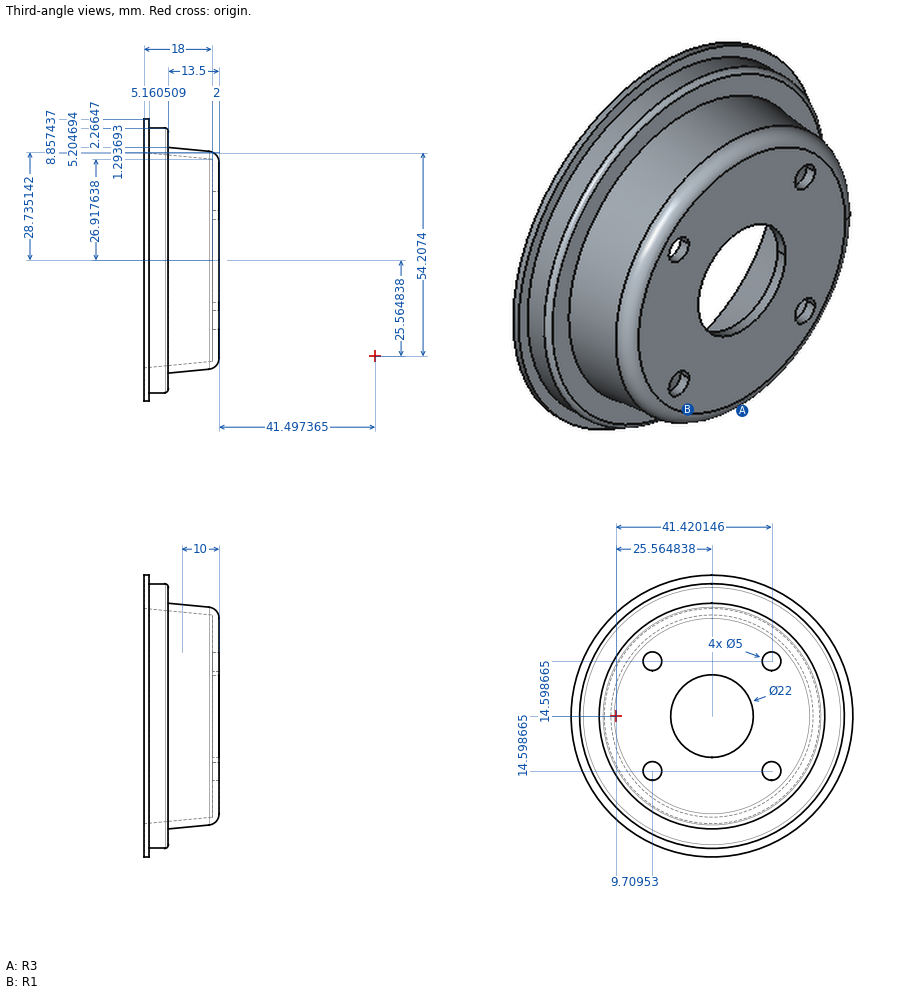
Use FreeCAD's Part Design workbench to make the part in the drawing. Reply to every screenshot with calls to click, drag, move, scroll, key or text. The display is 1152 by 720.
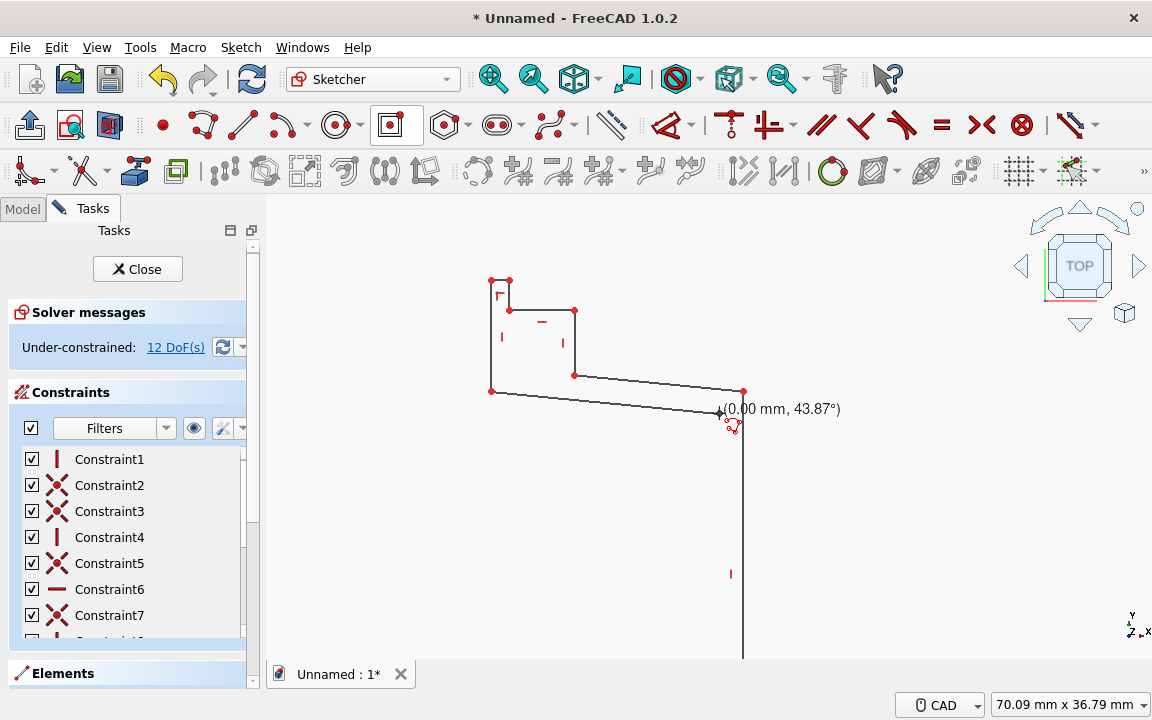
scroll(501, 280, down, 5)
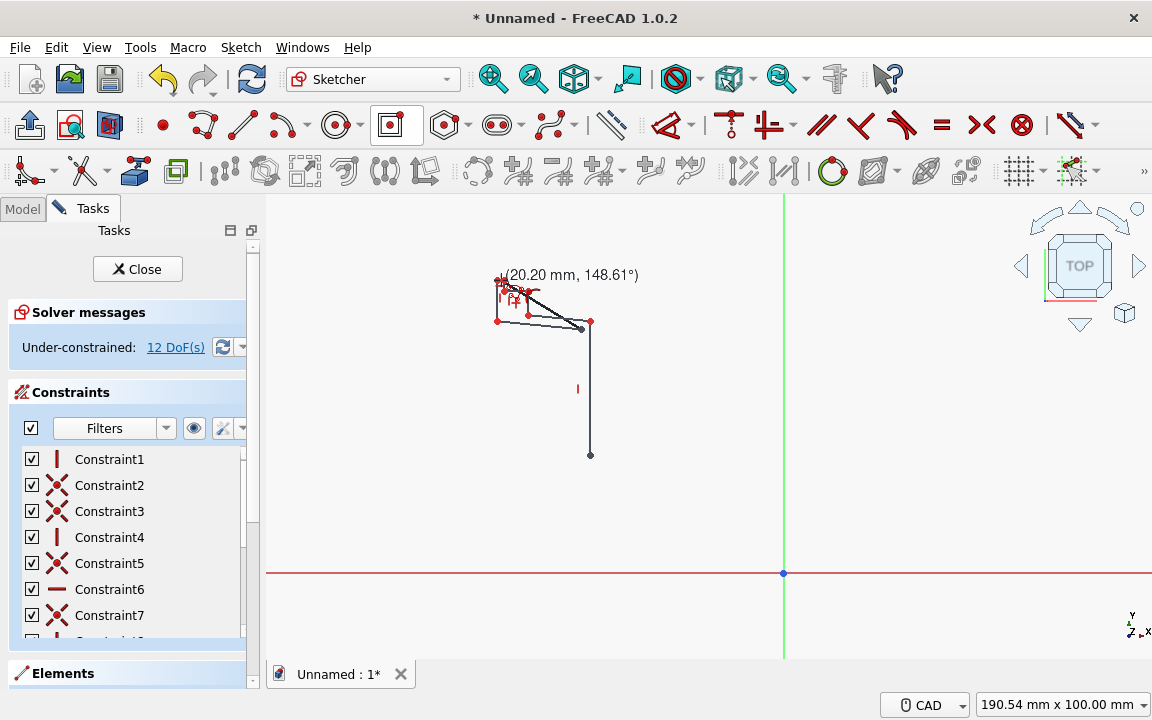
scroll(581, 454, up, 3)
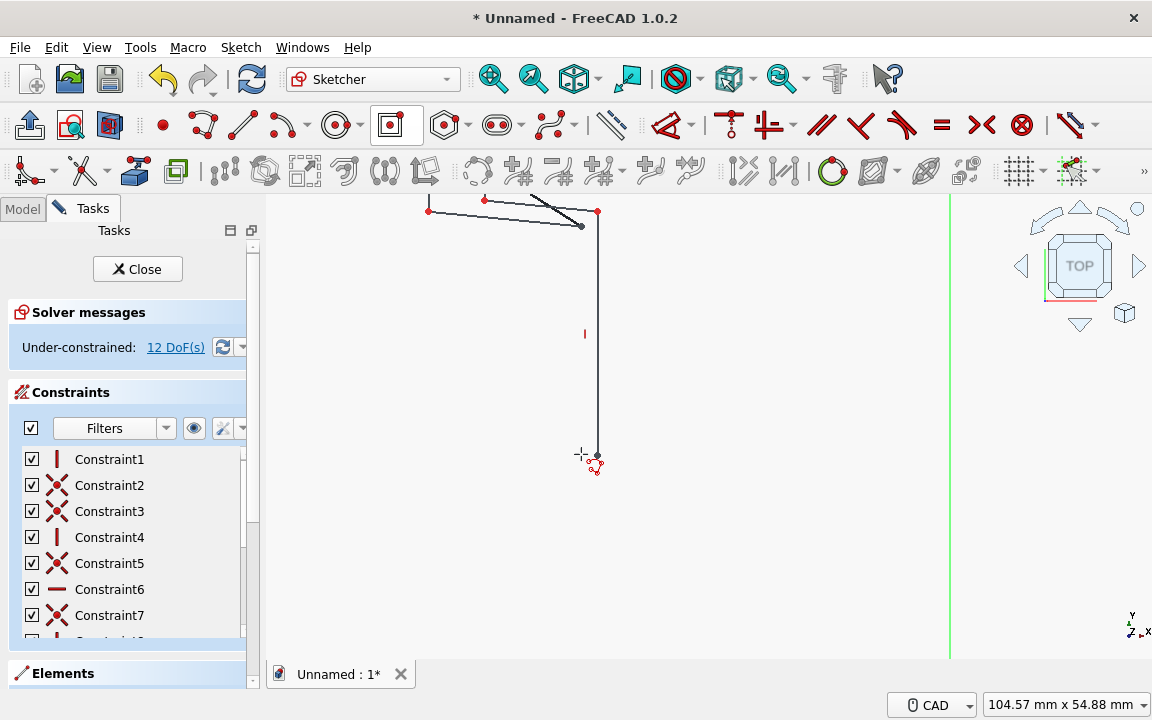
click(581, 454)
click(598, 456)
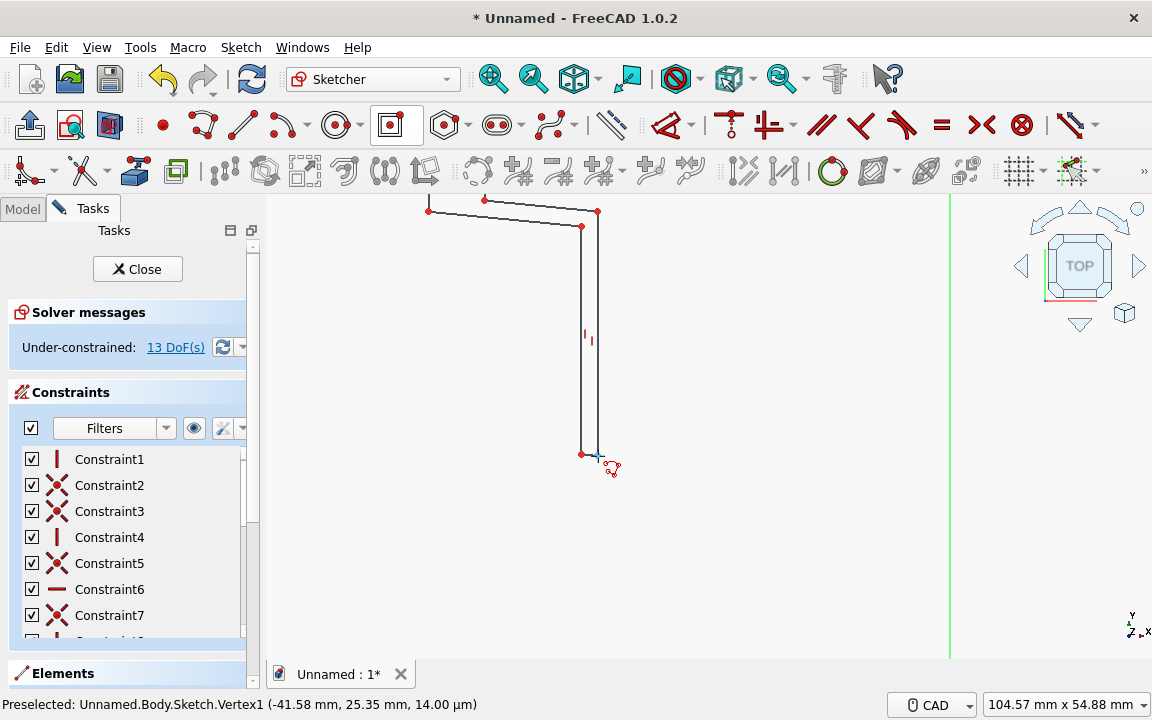
click(244, 126)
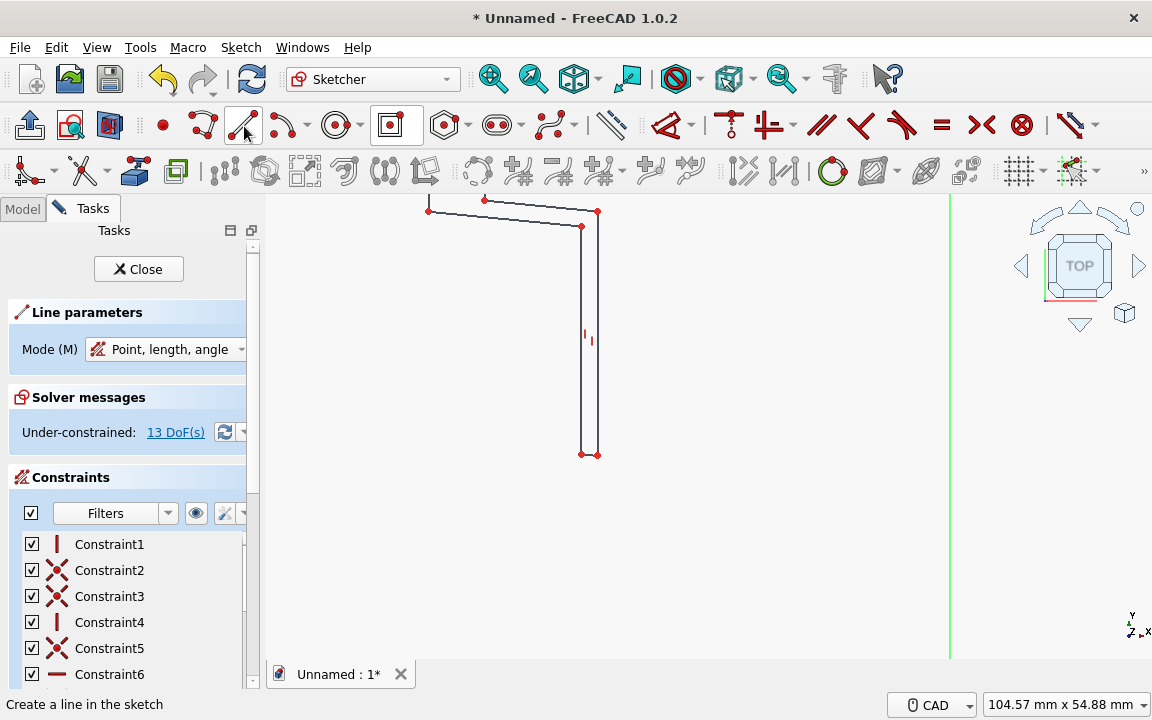
click(615, 454)
click(666, 454)
key(Escape)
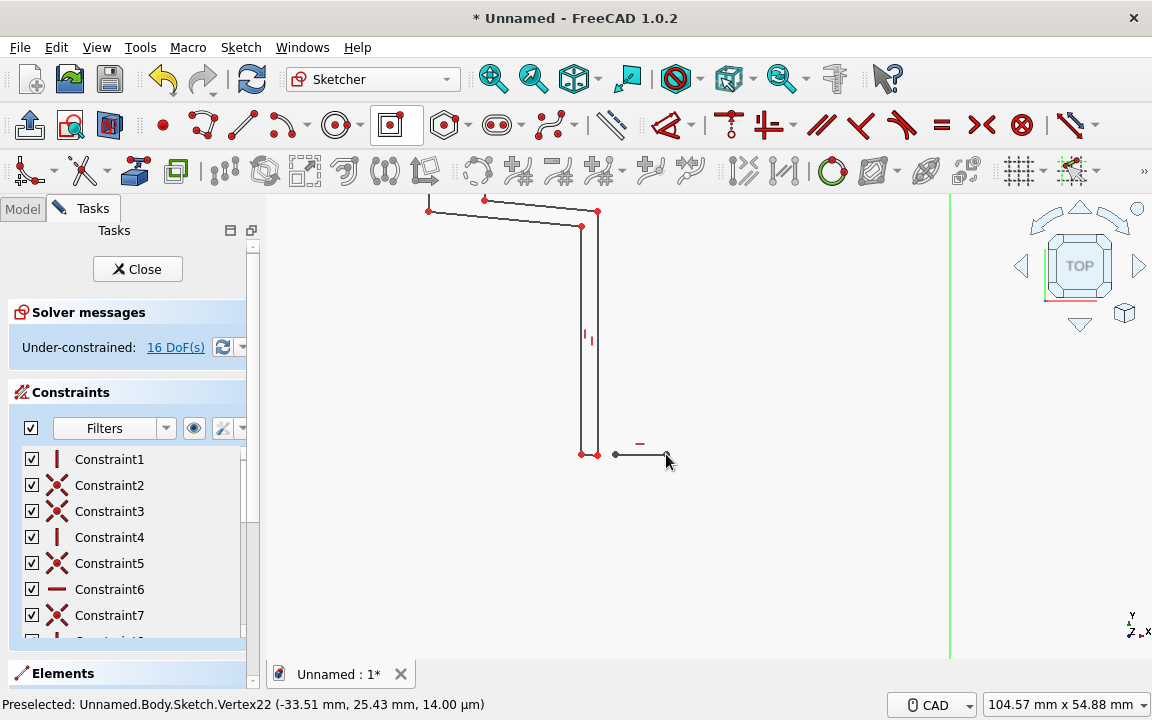
click(630, 455)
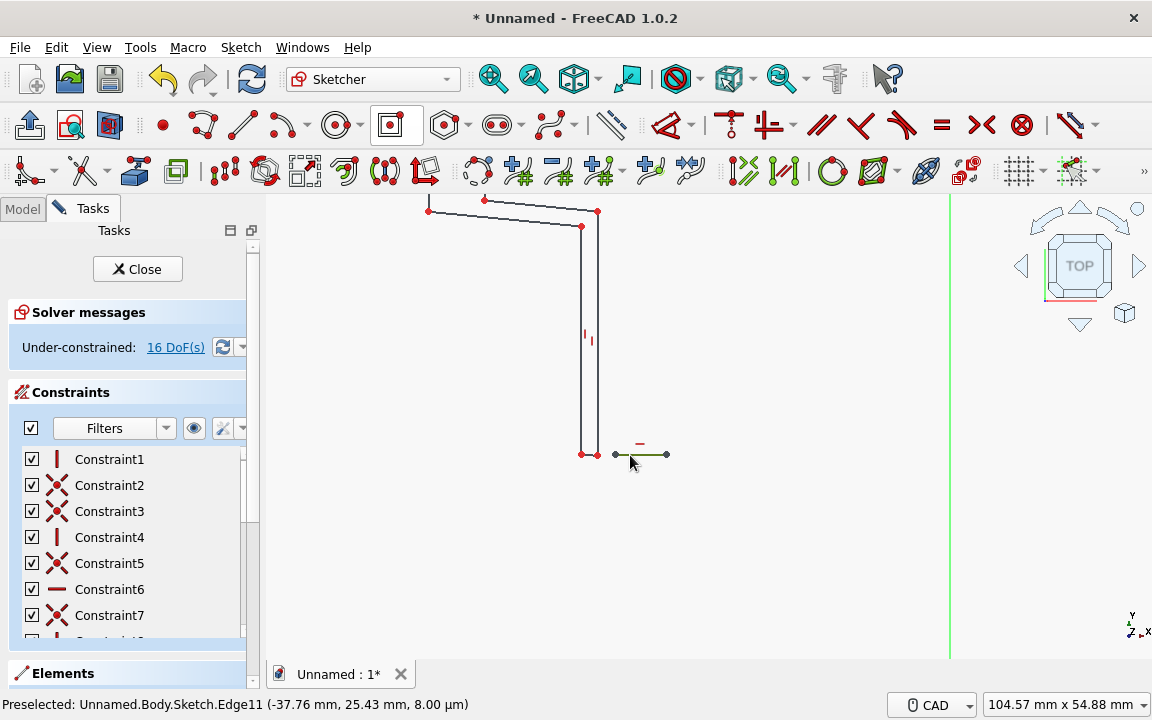
key(g)
key(n)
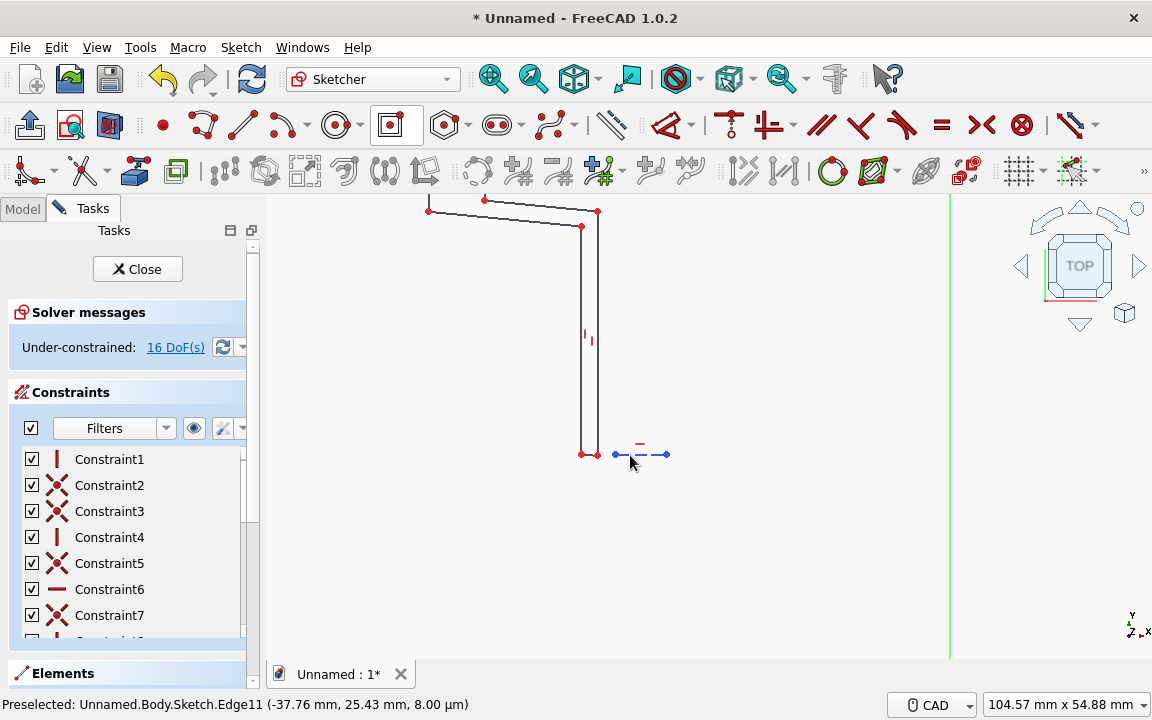
scroll(589, 455, up, 3)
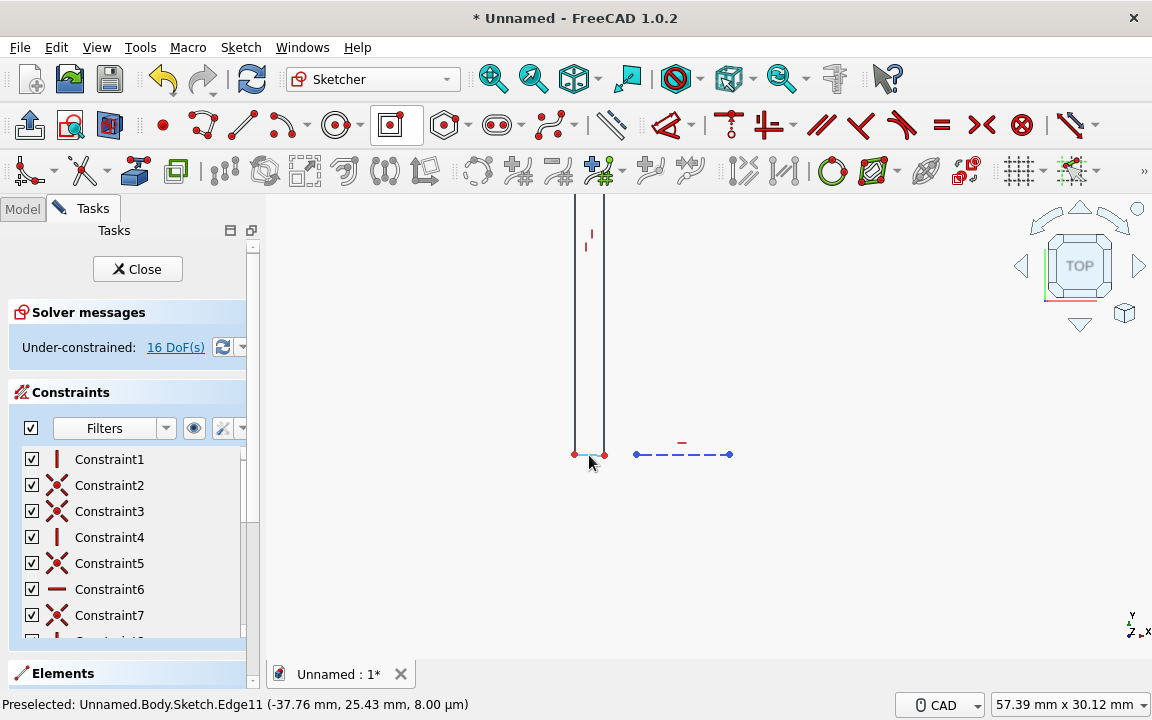
click(590, 455)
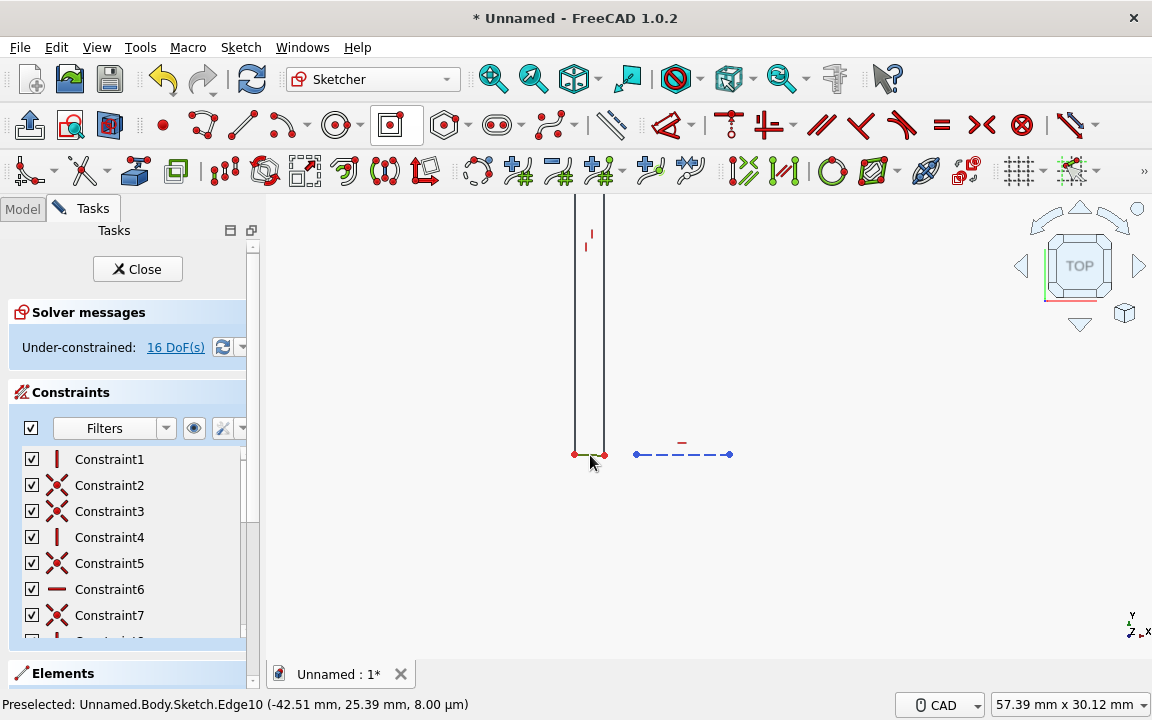
key(h)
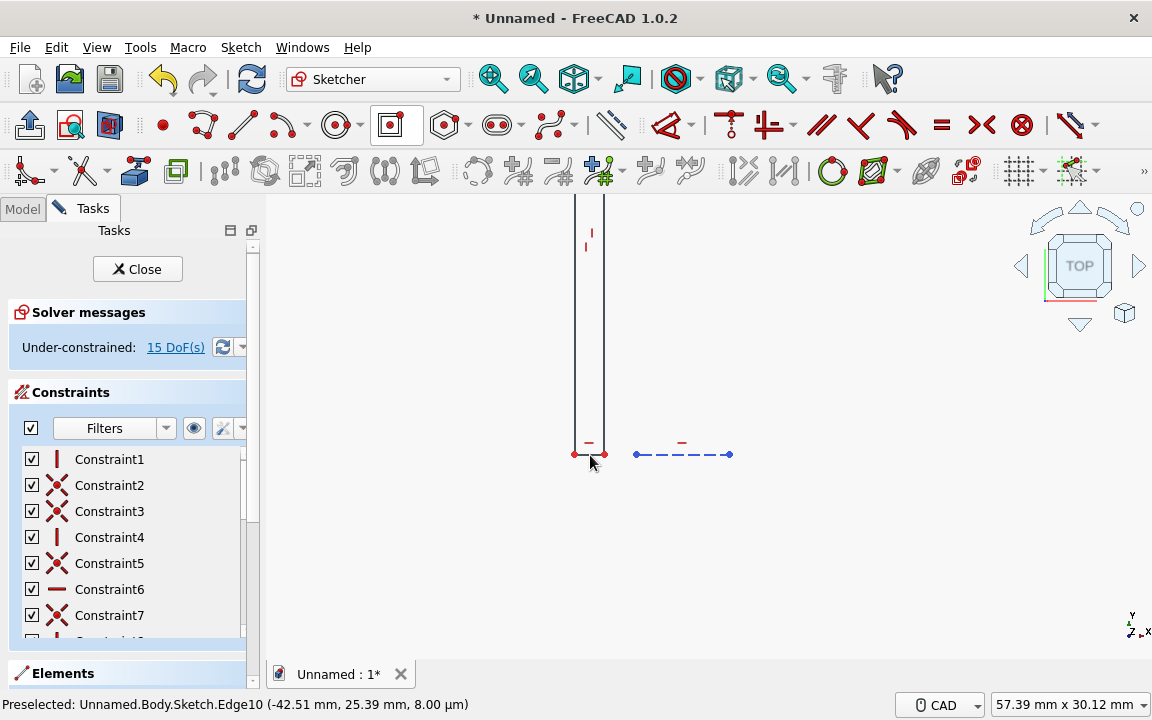
scroll(587, 455, up, 2)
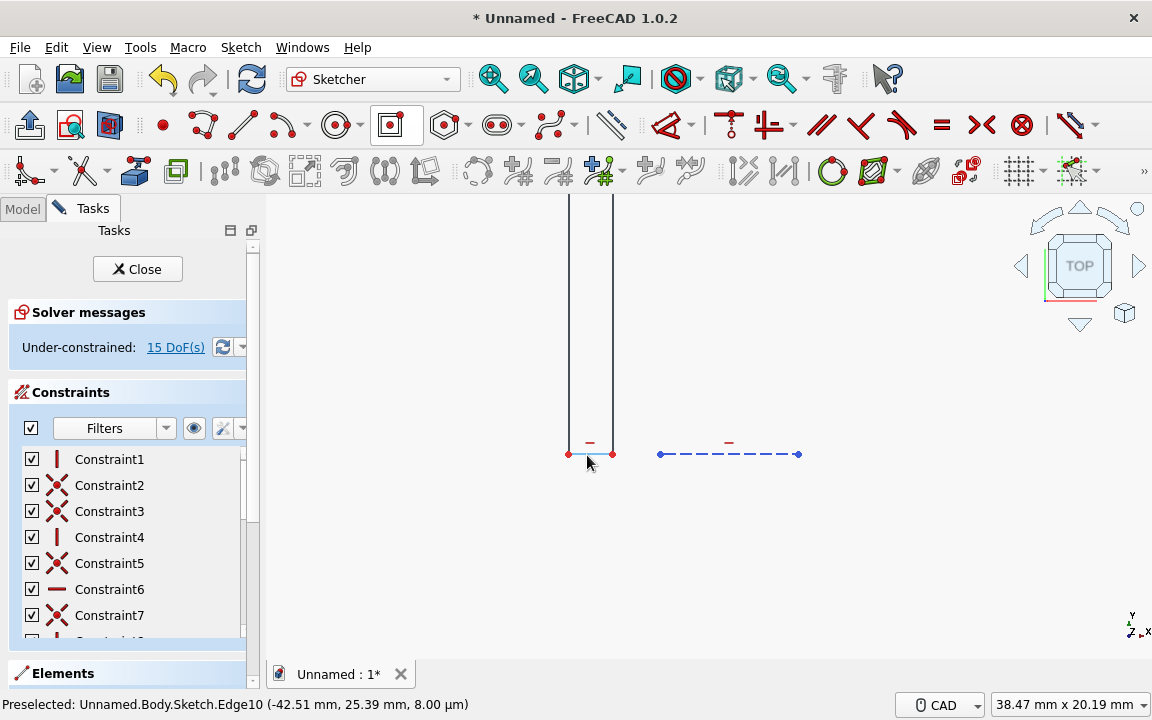
click(586, 454)